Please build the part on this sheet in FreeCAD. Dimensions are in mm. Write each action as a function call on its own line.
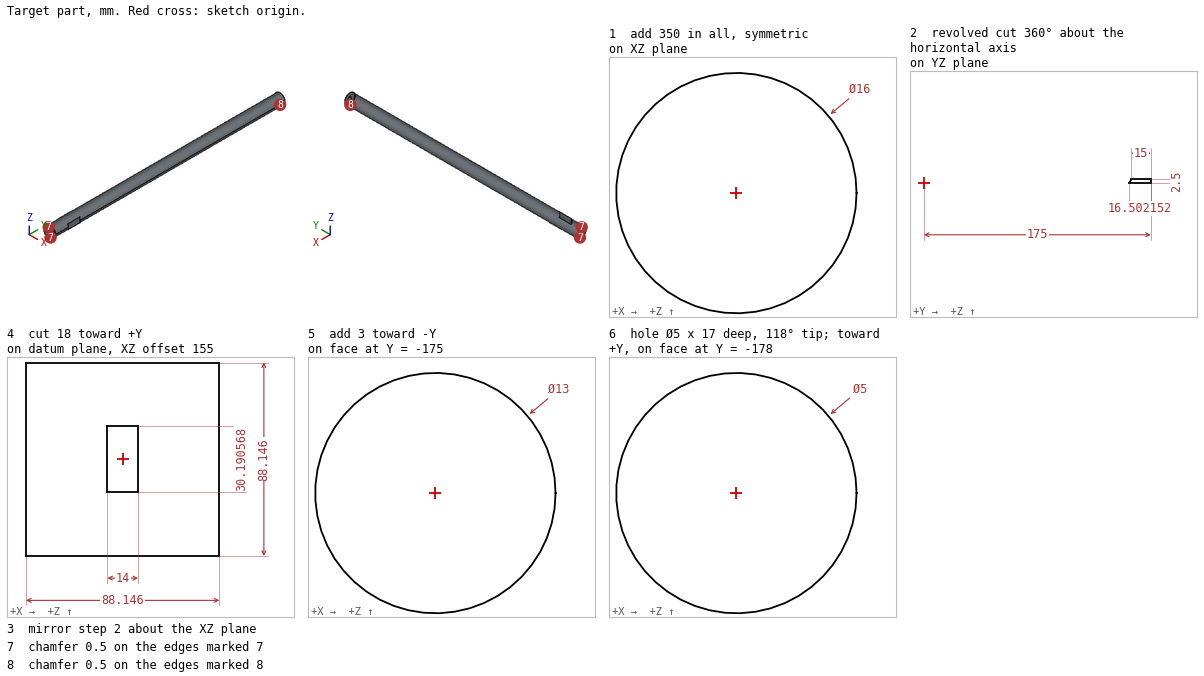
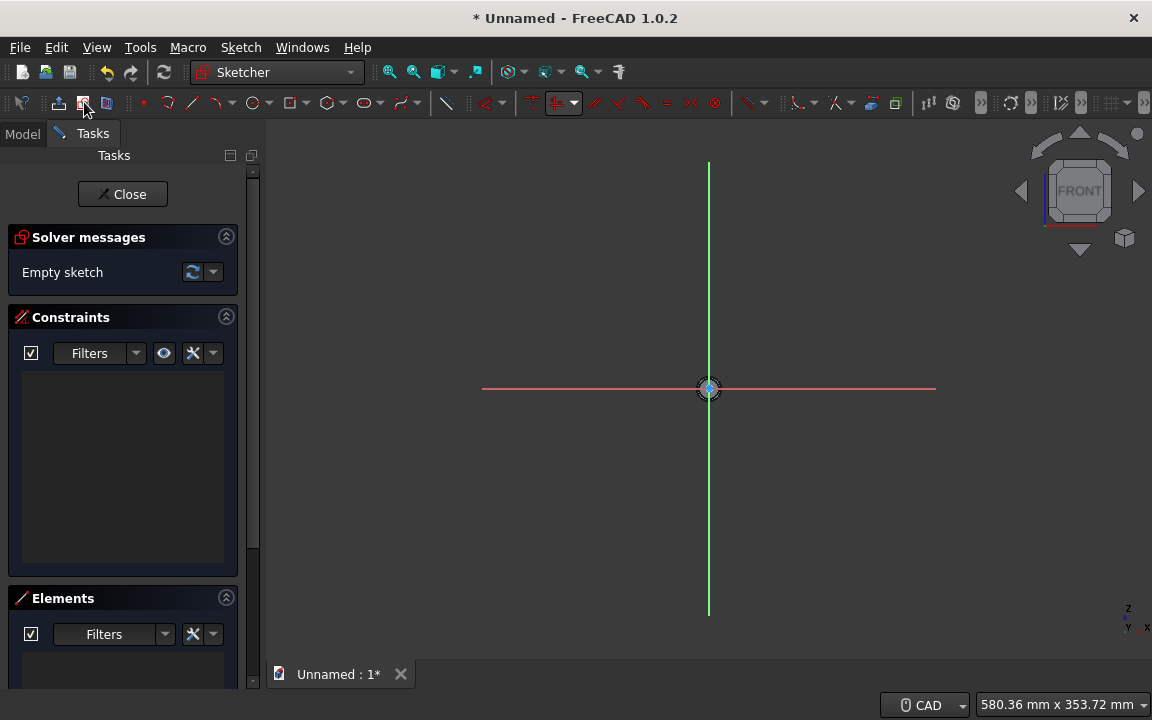
scroll(713, 389, up, 15)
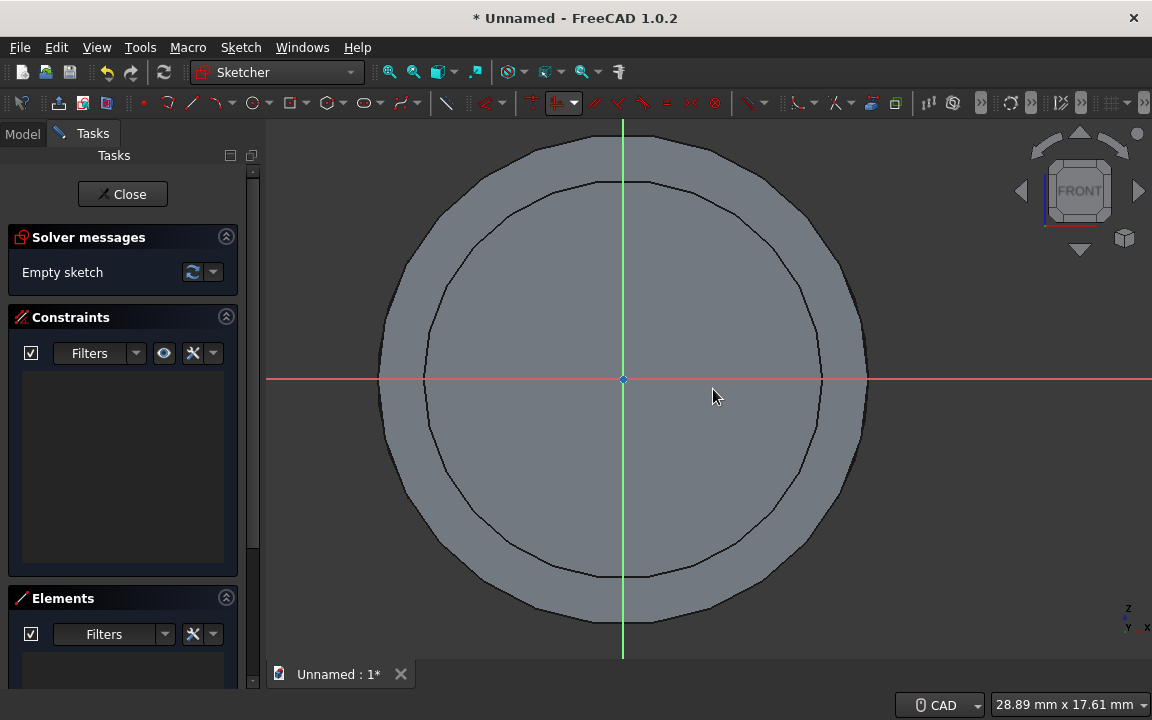
scroll(609, 372, up, 4)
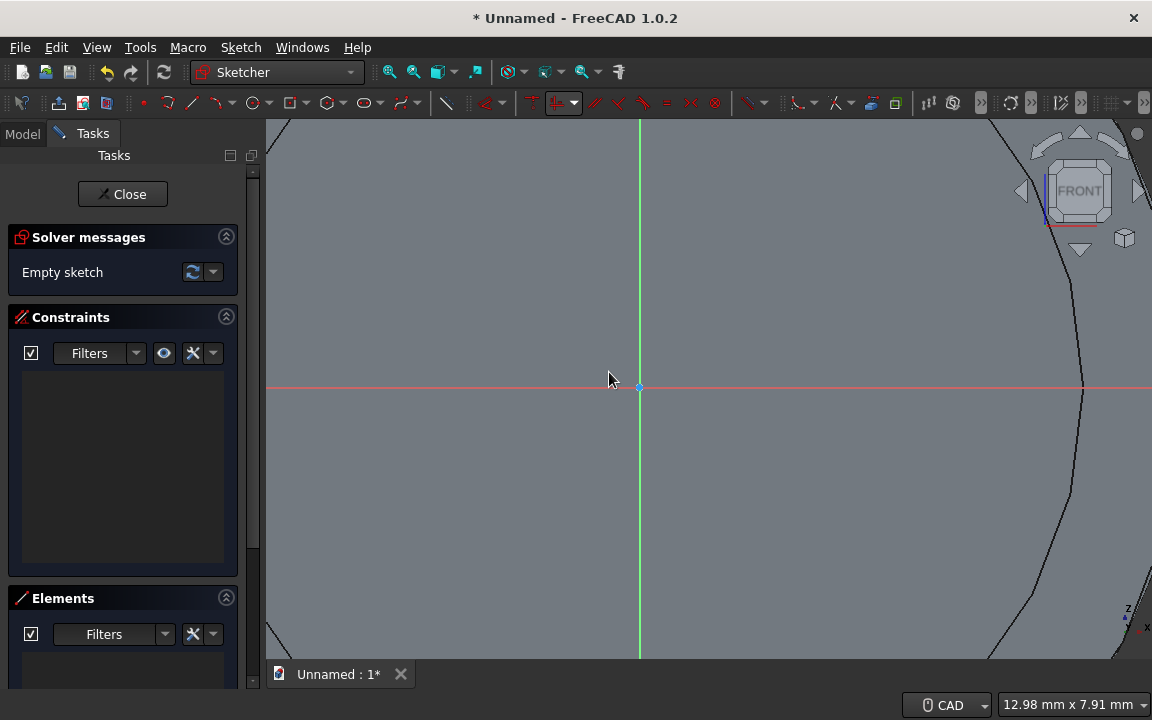
click(254, 104)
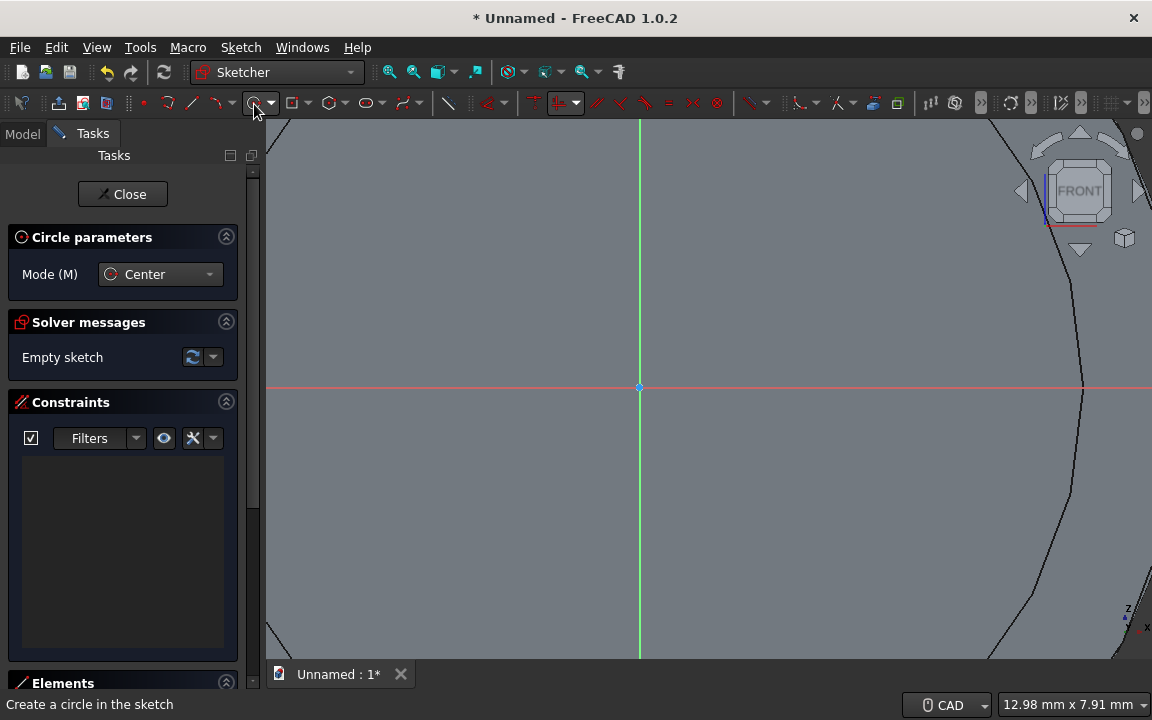
click(640, 388)
move(760, 267)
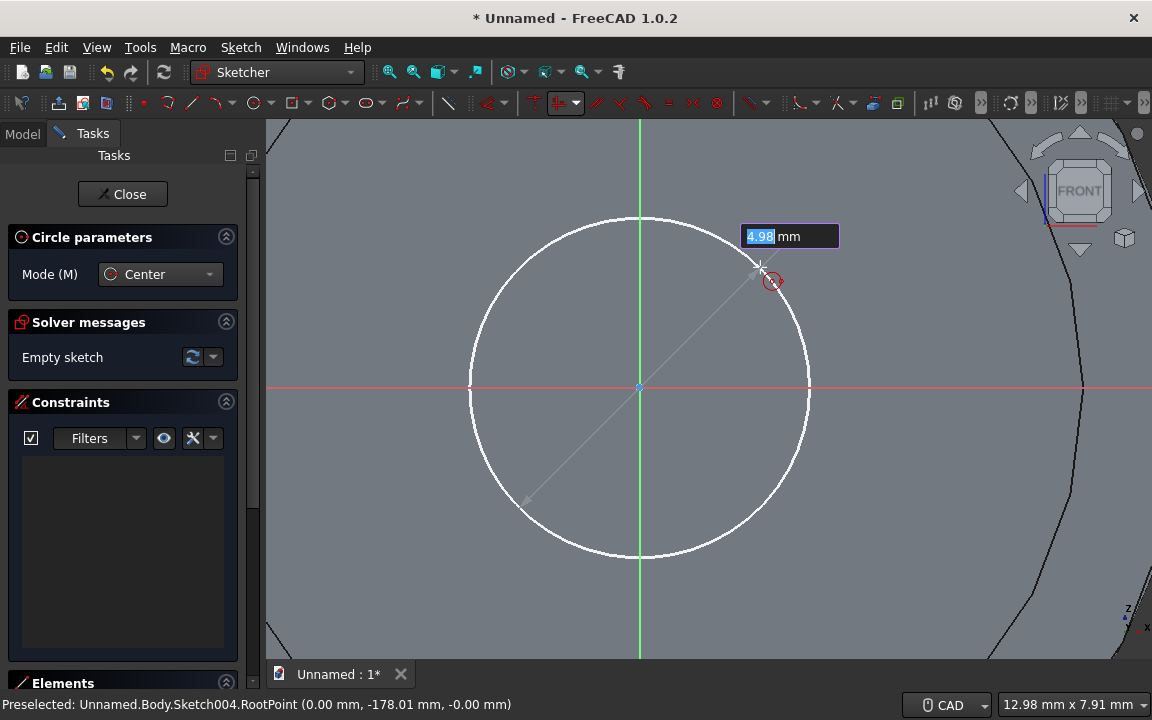
text(5)
key(Return)
key(Escape)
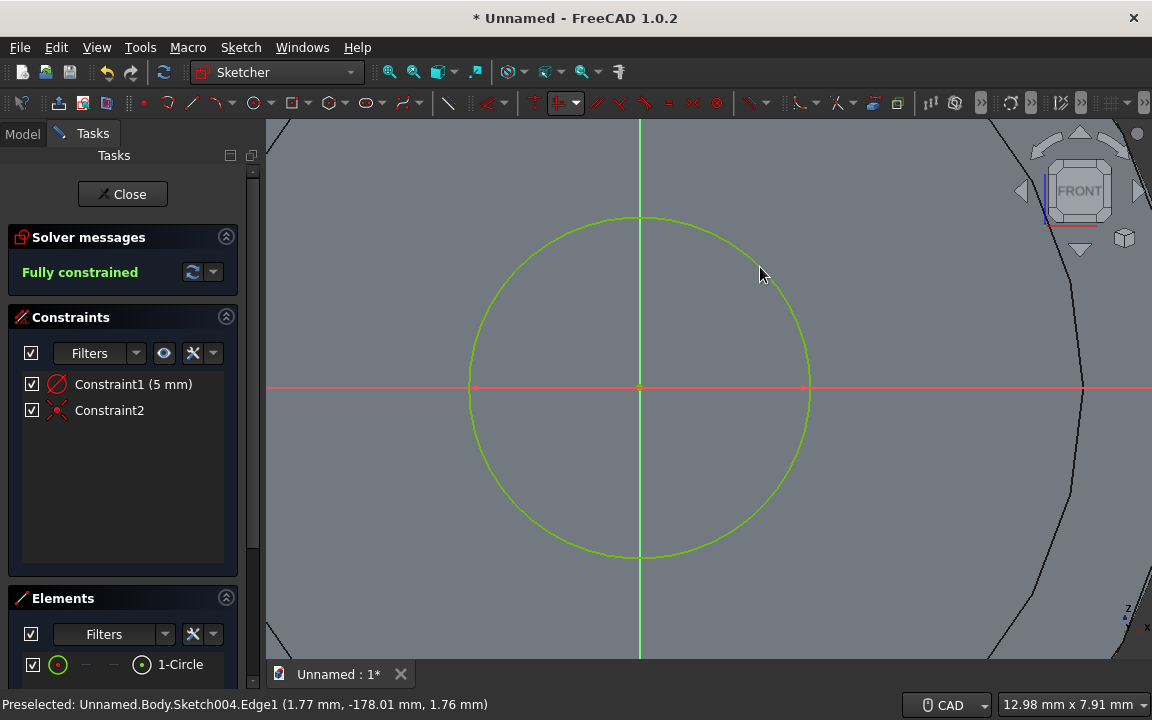
click(123, 194)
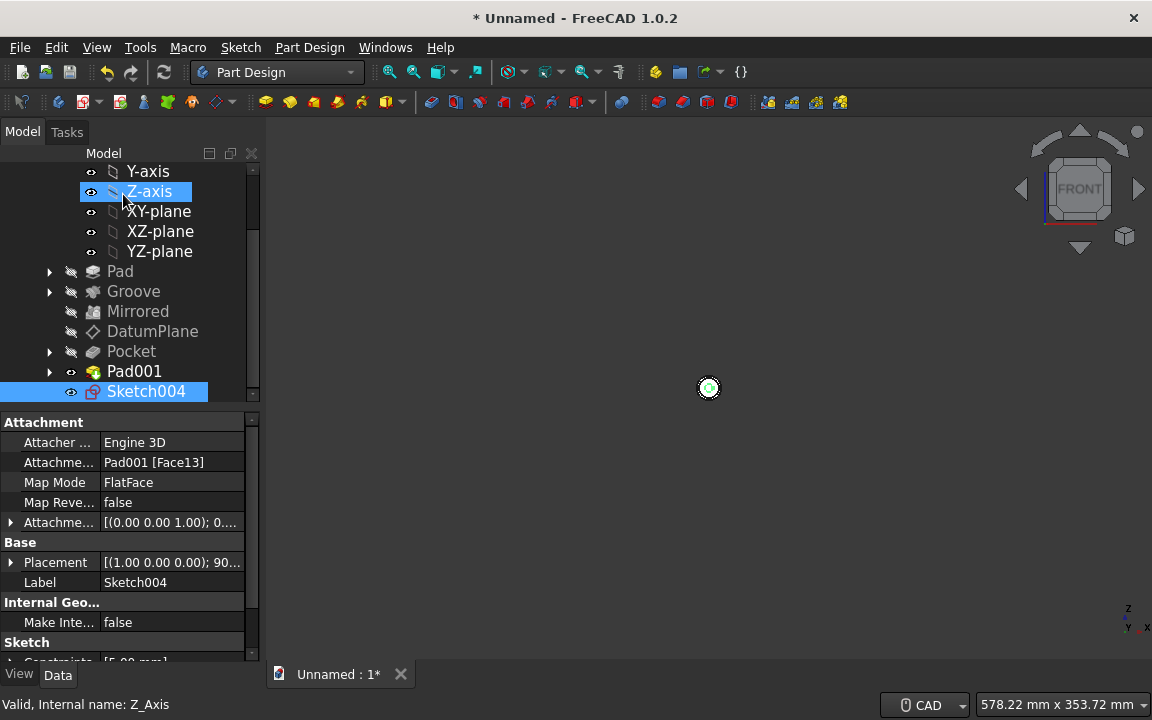
click(456, 102)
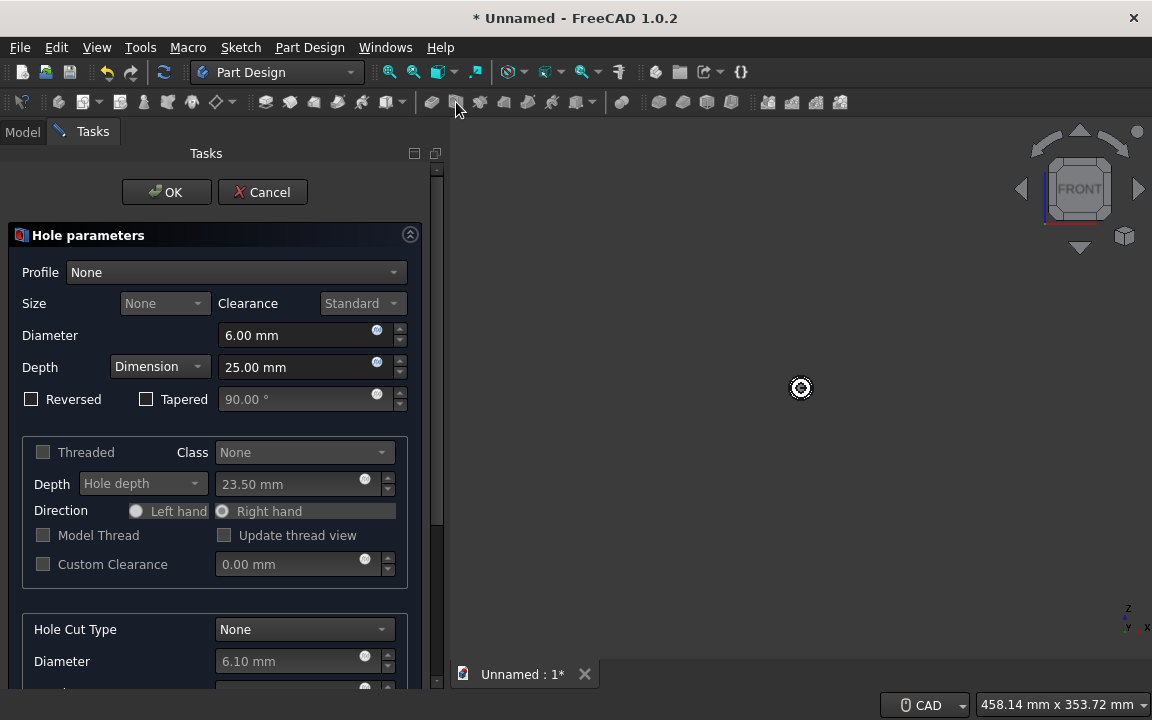
triple_click(305, 335)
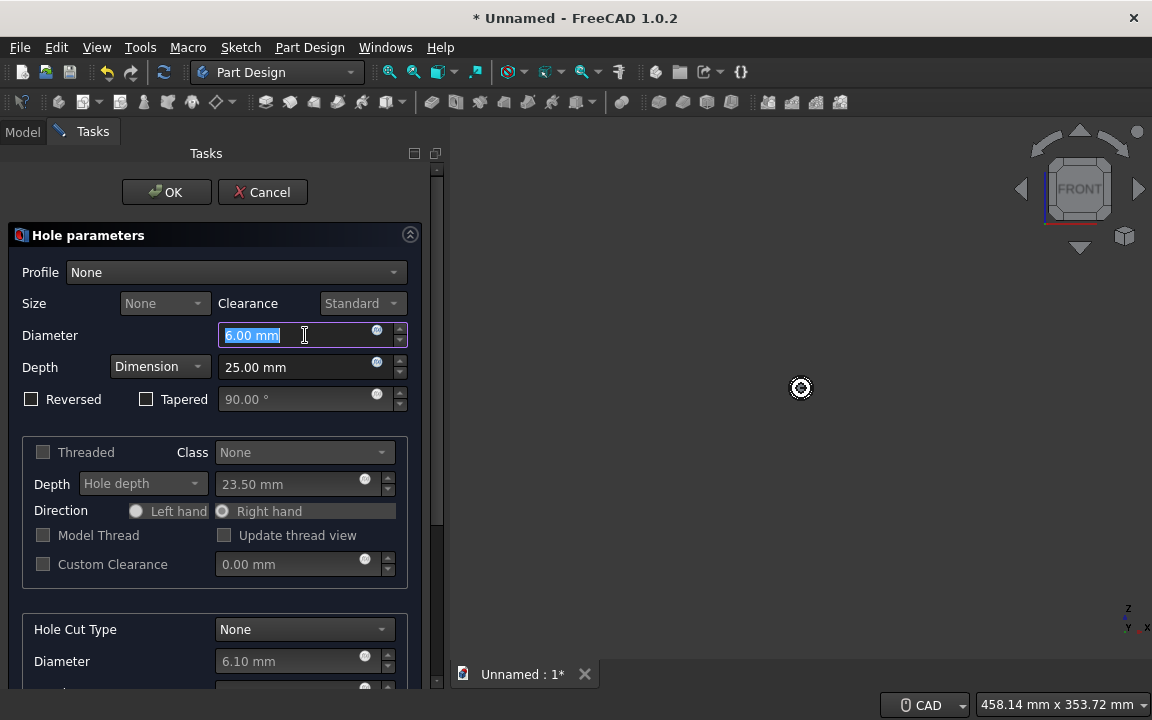
text(5)
key(Tab)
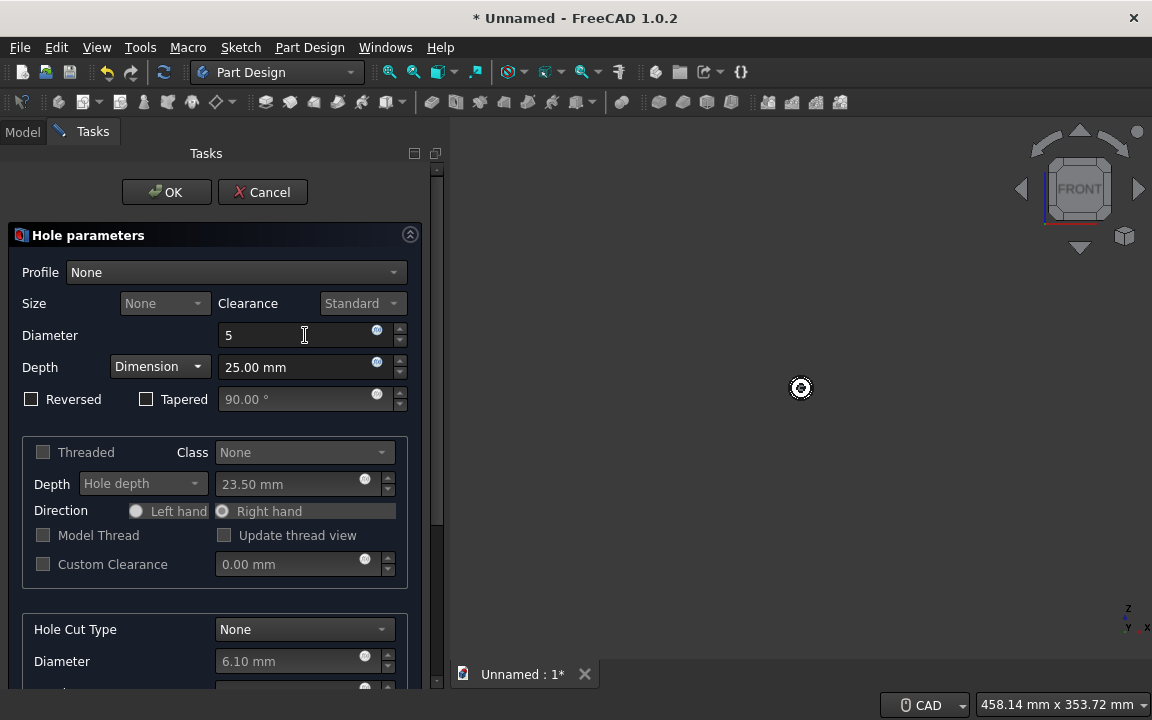
triple_click(305, 367)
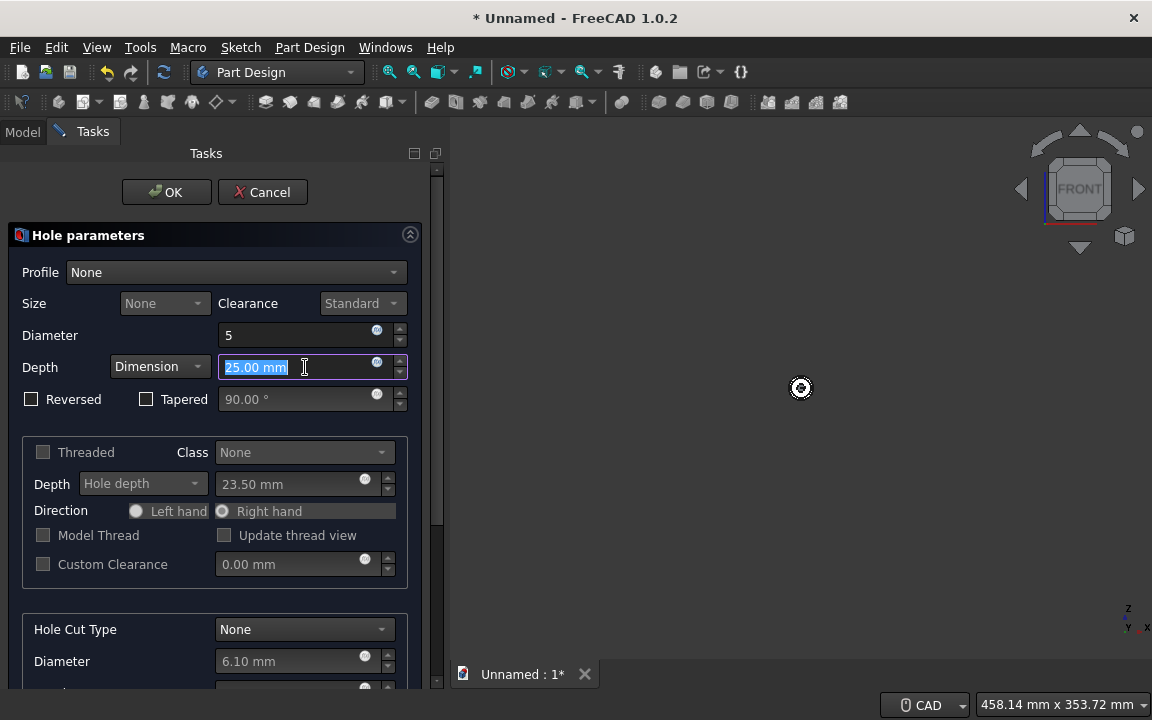
text(17)
key(Tab)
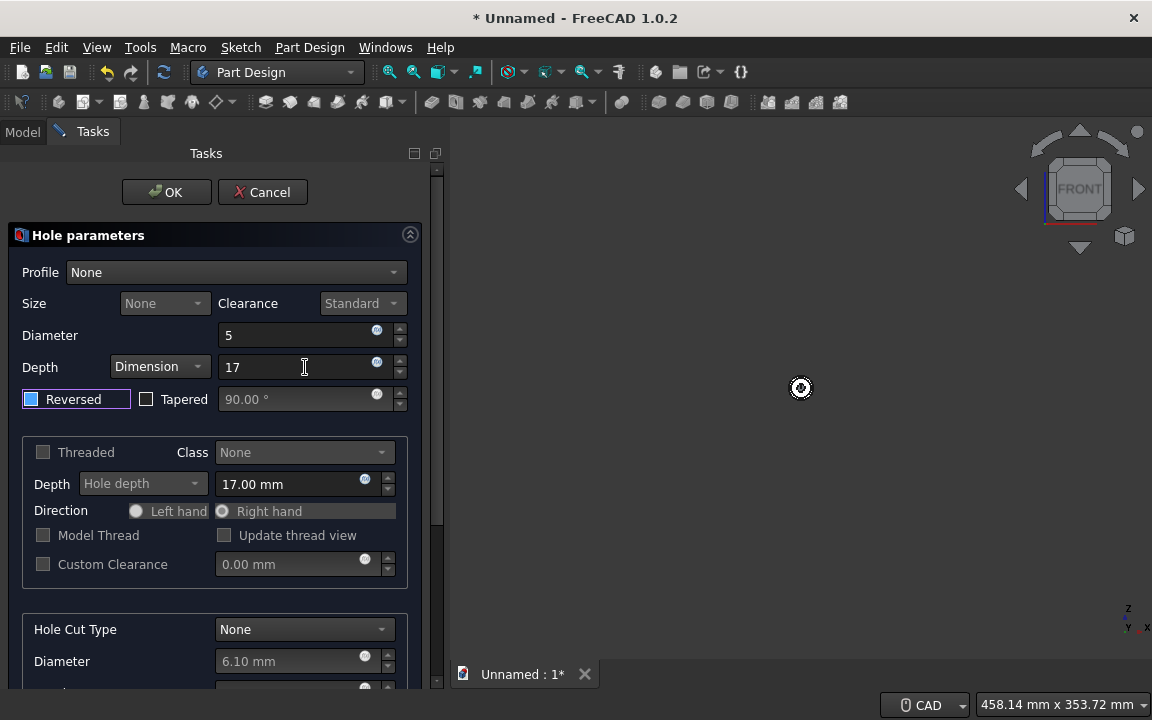
click(167, 192)